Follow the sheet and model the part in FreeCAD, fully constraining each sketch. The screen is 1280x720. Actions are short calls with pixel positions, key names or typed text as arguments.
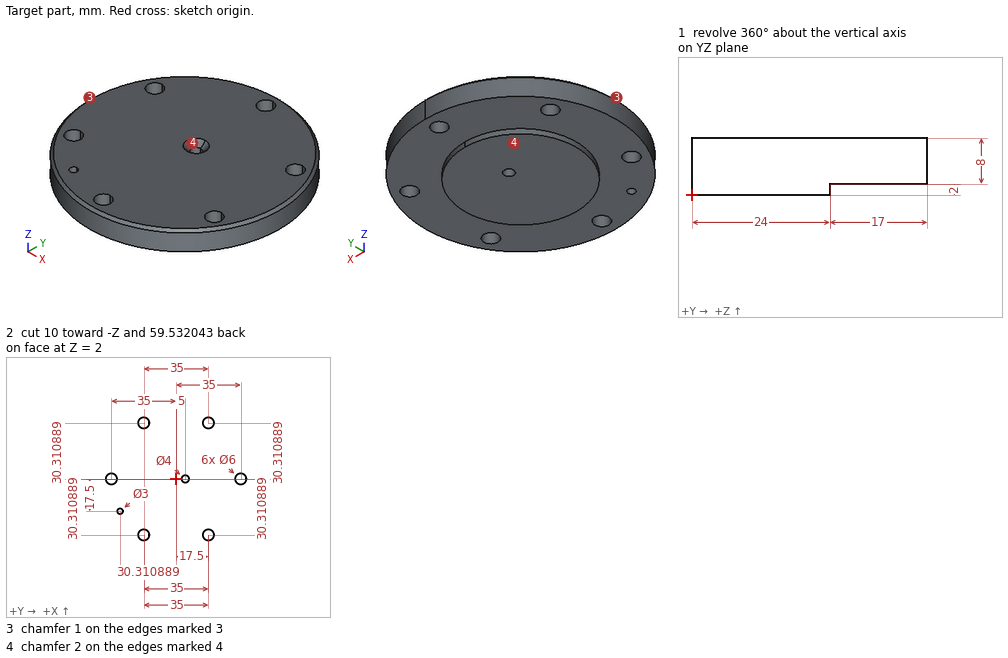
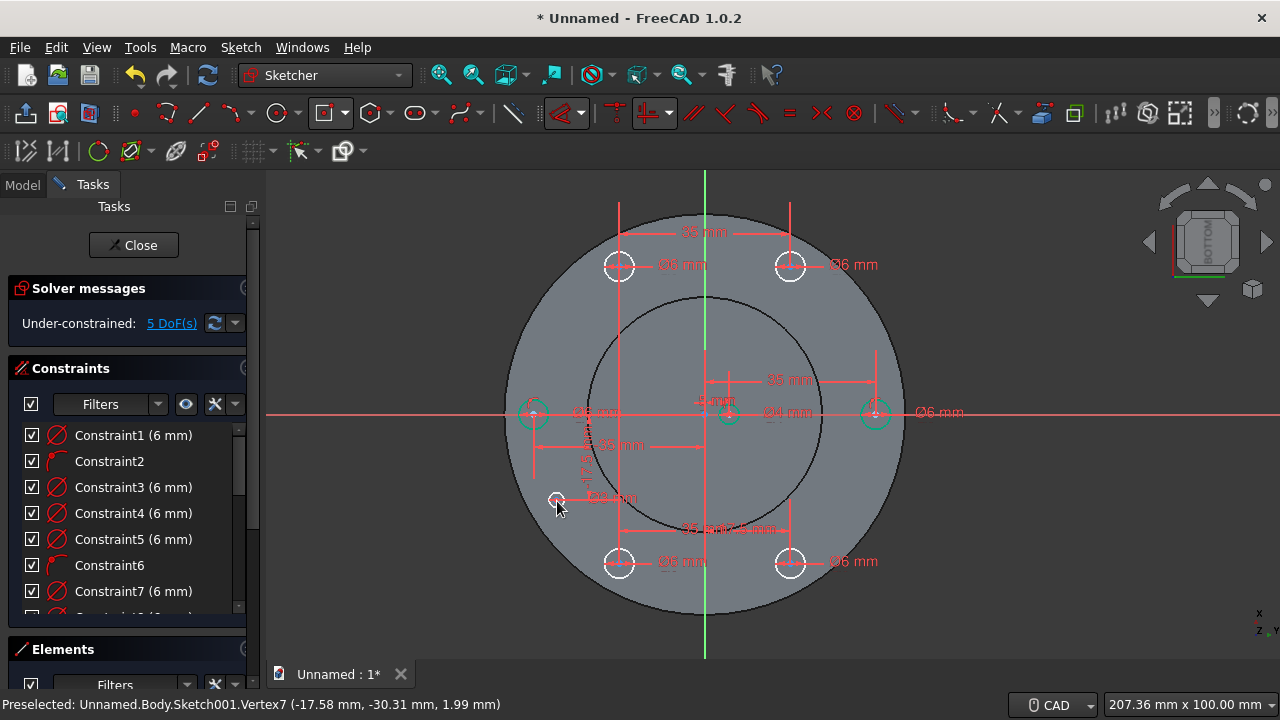
click(790, 564)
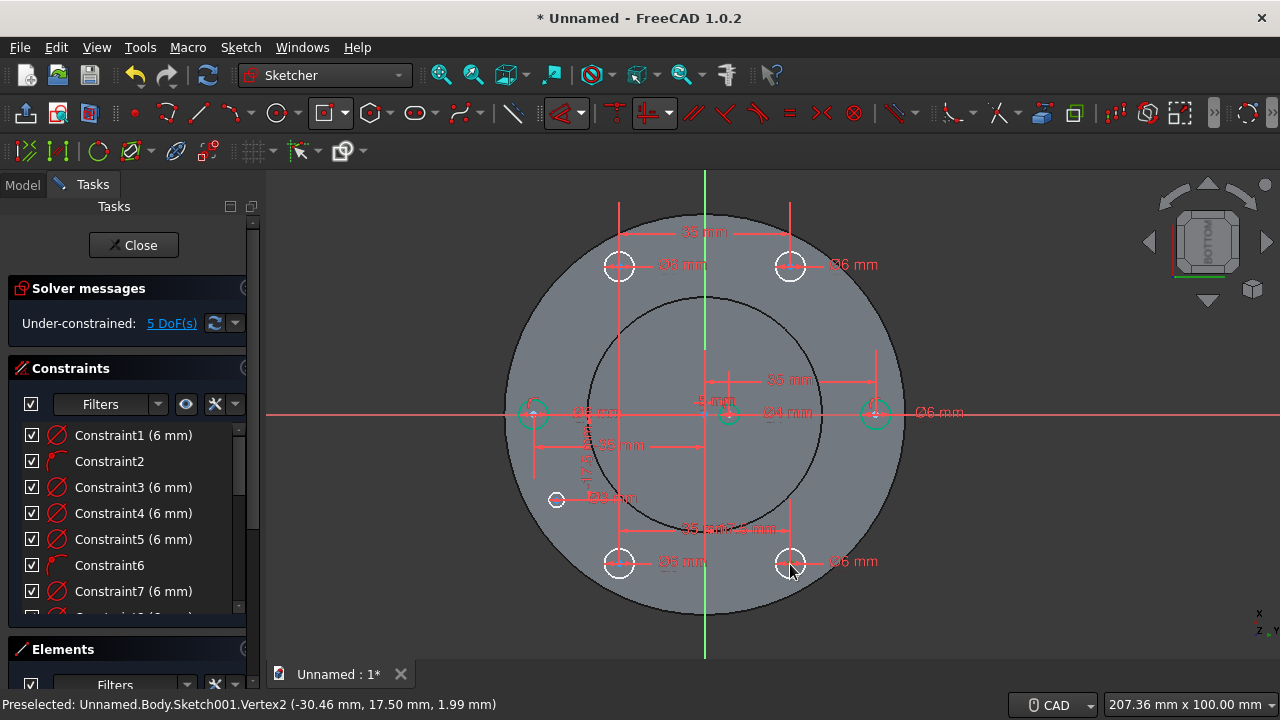
key(i)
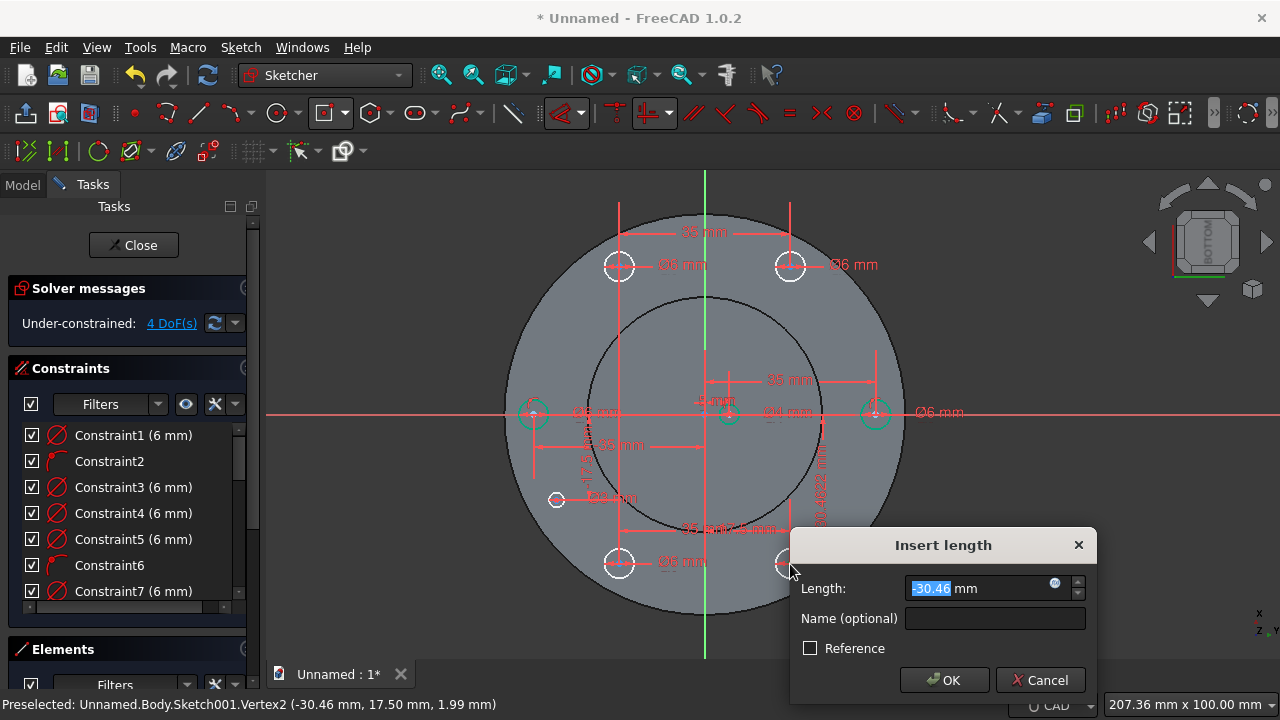
text(-30.310889)
key(Return)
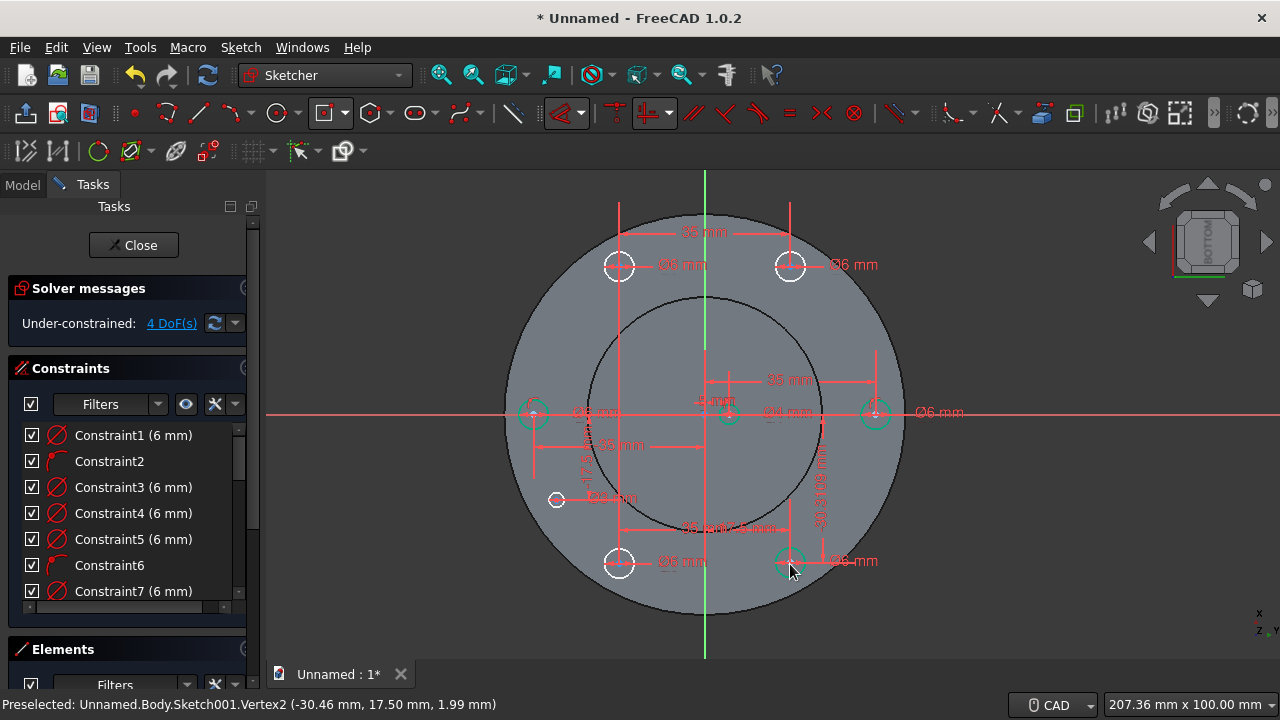
click(619, 564)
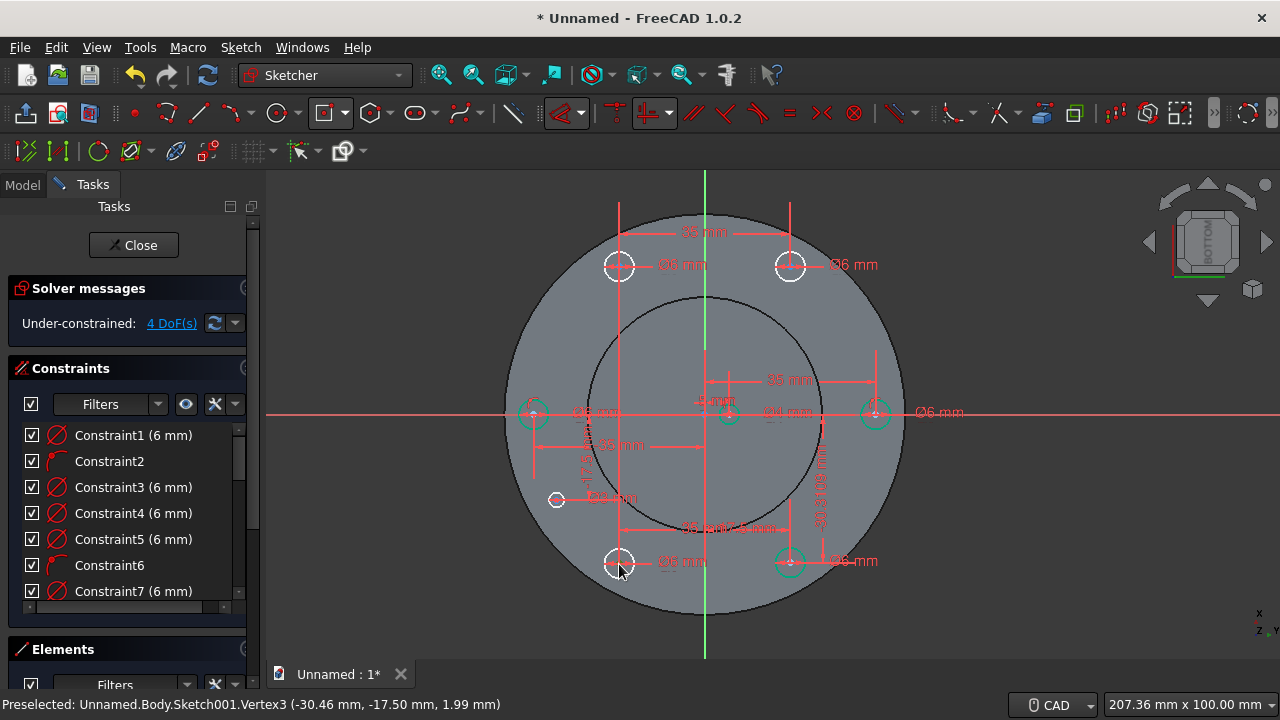
key(i)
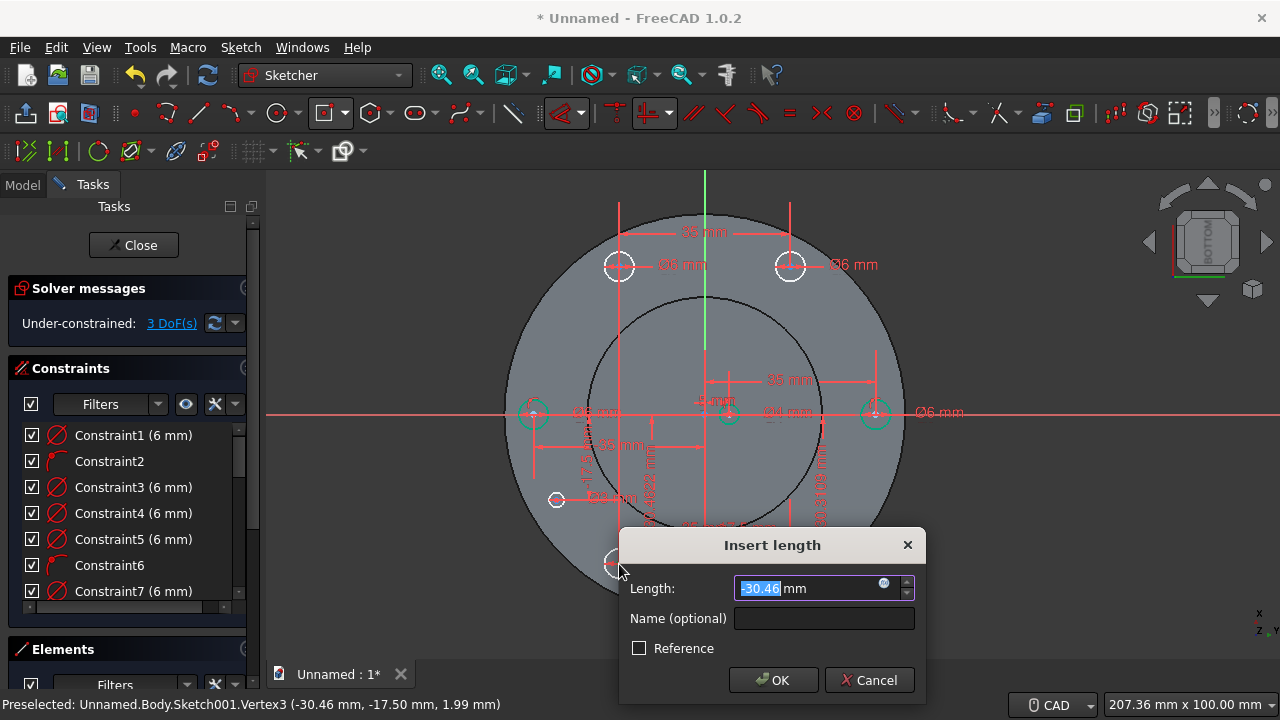
text(-30.310889)
key(Return)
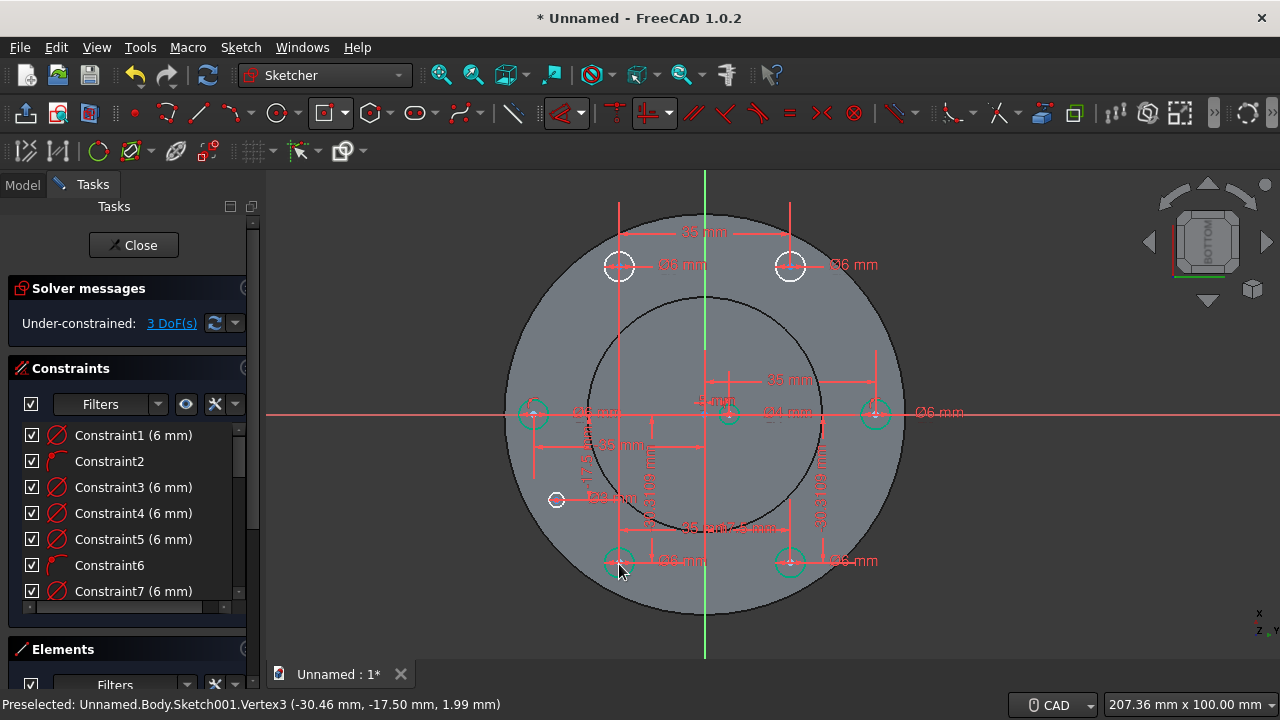
click(619, 267)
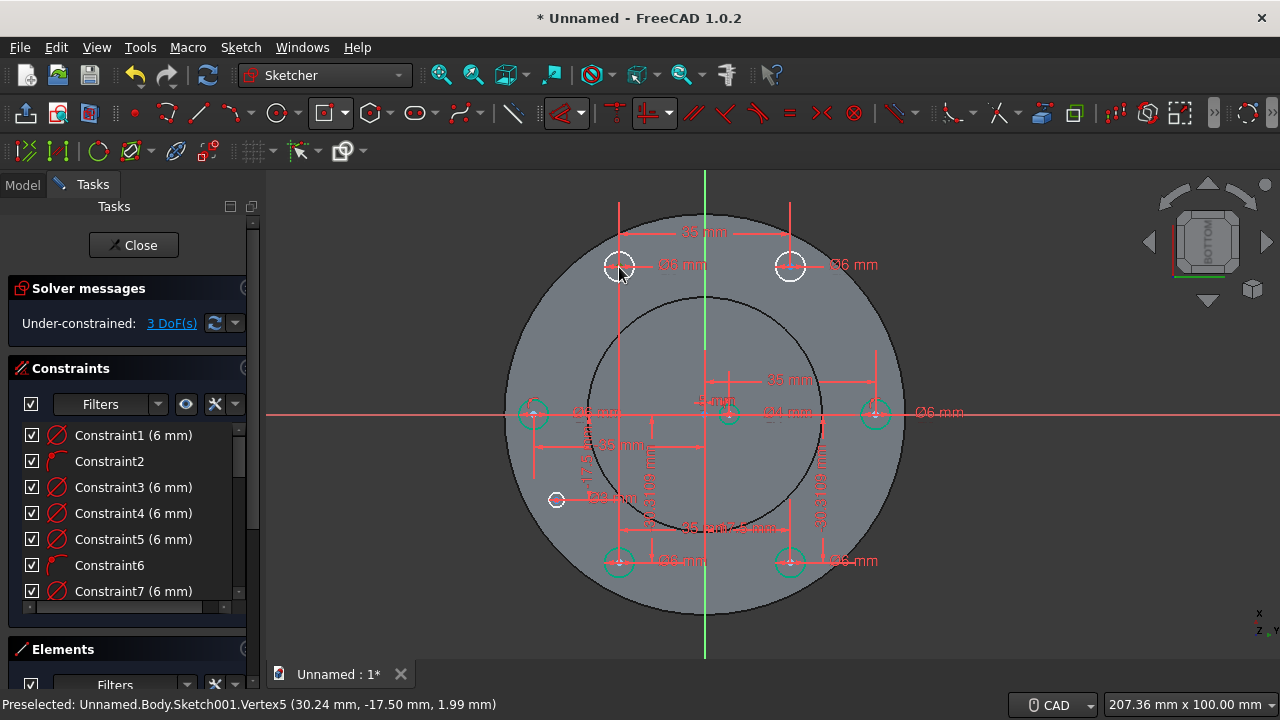
key(i)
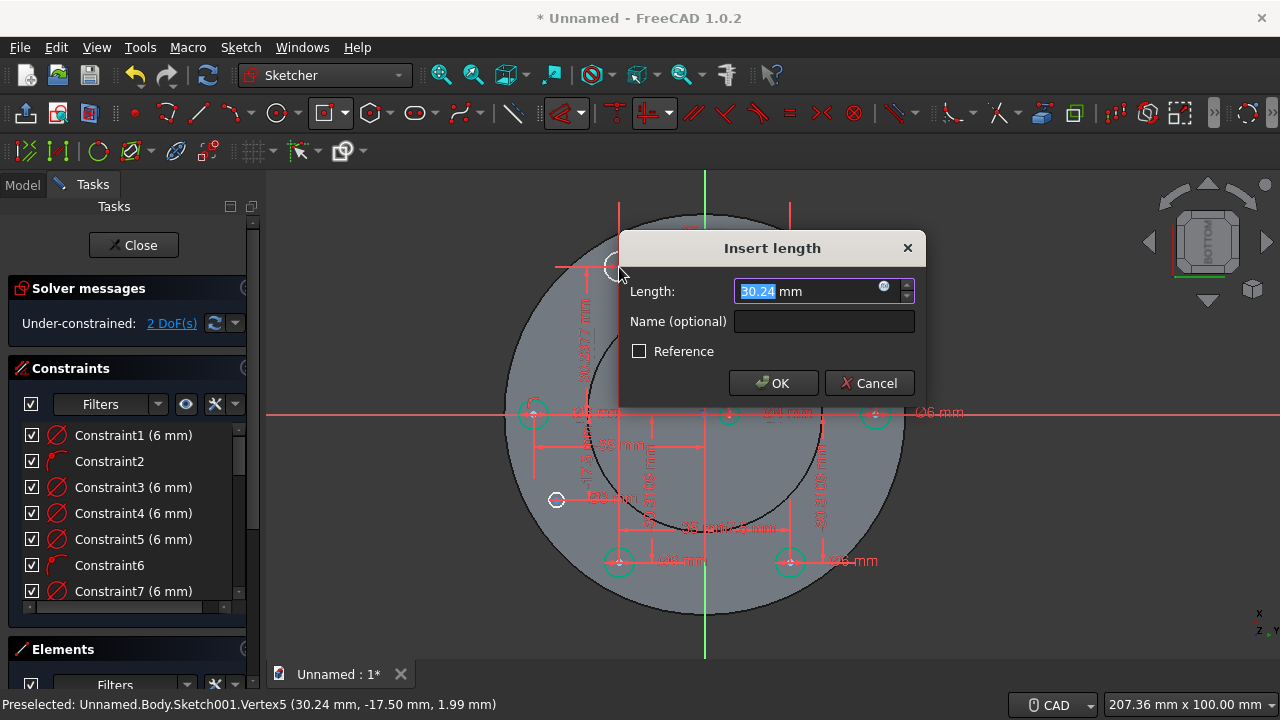
text(30.310889)
key(Return)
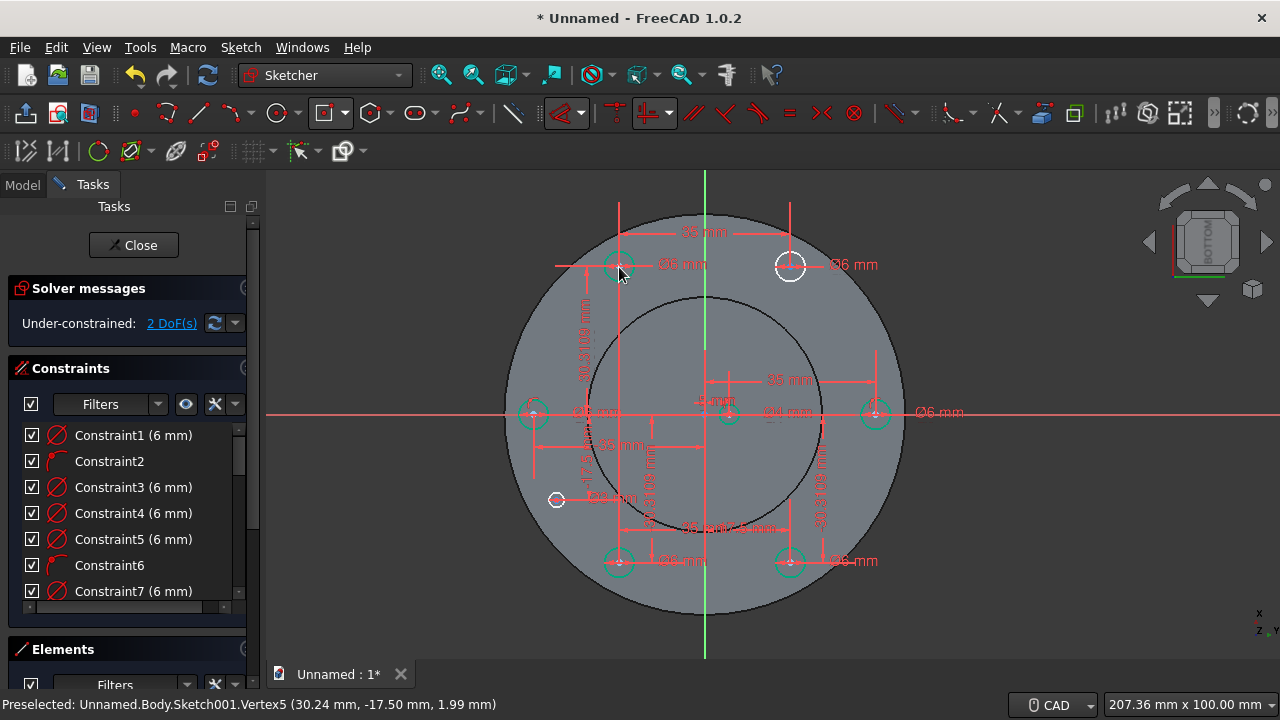
click(790, 267)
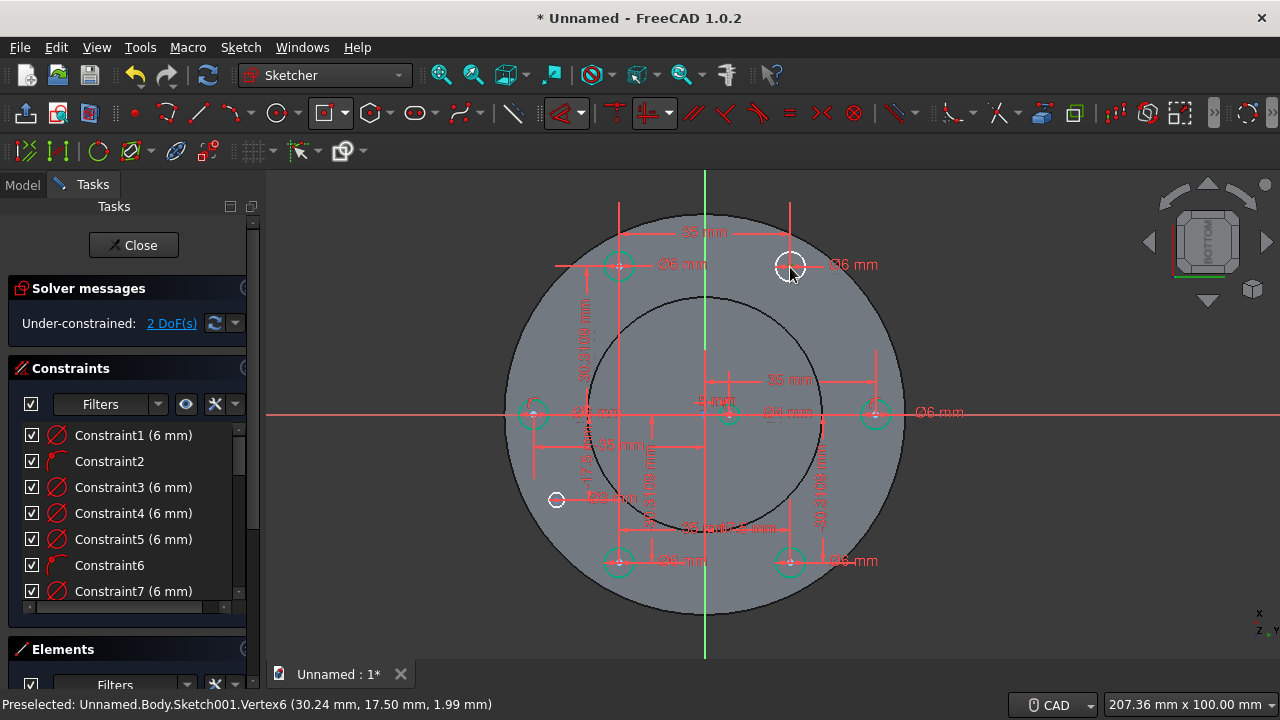
key(i)